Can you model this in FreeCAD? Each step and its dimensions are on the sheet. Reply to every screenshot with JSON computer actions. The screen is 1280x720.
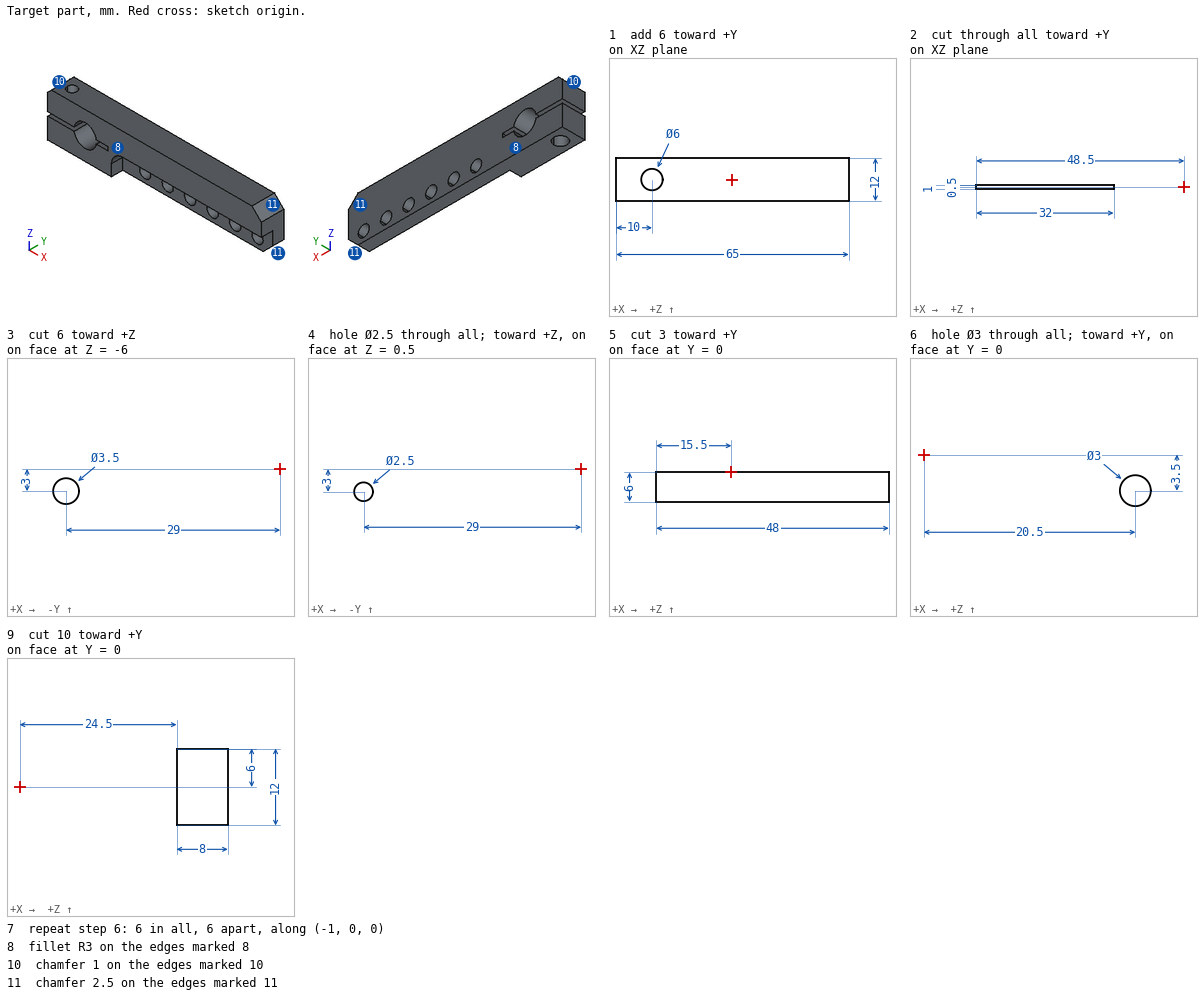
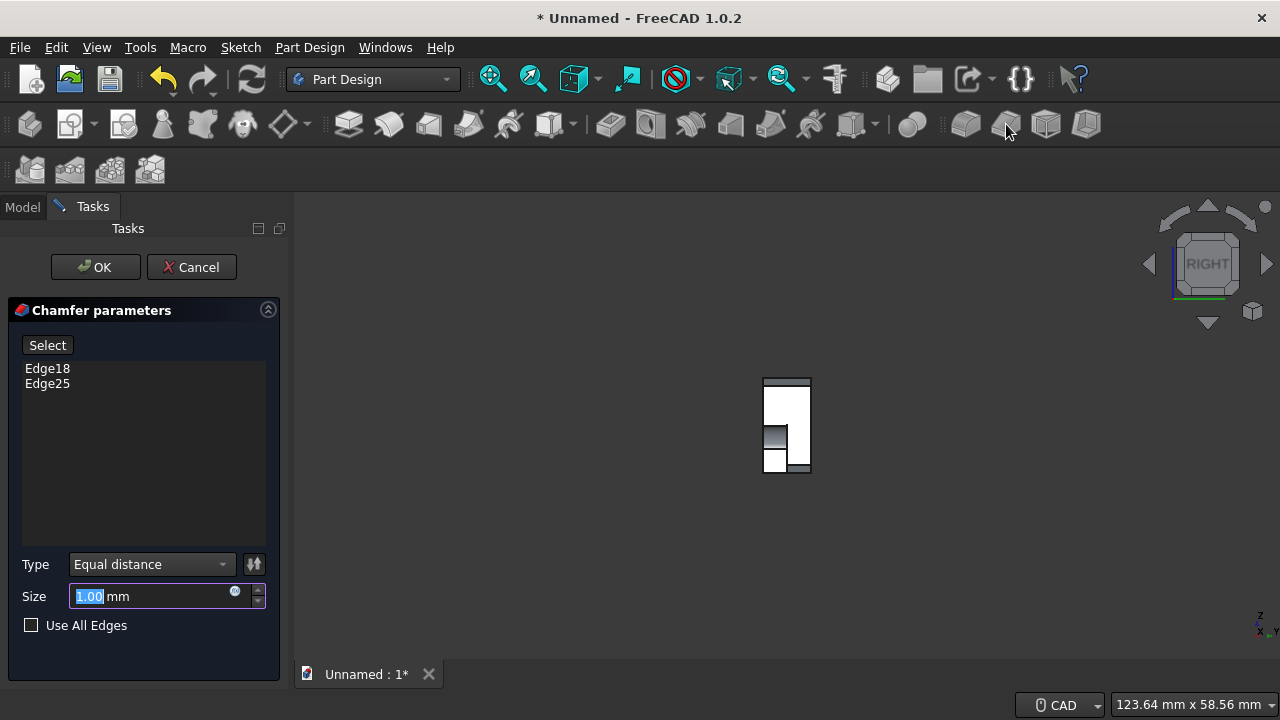
{"action": "type", "text": "2.5"}
{"action": "key", "text": "Tab"}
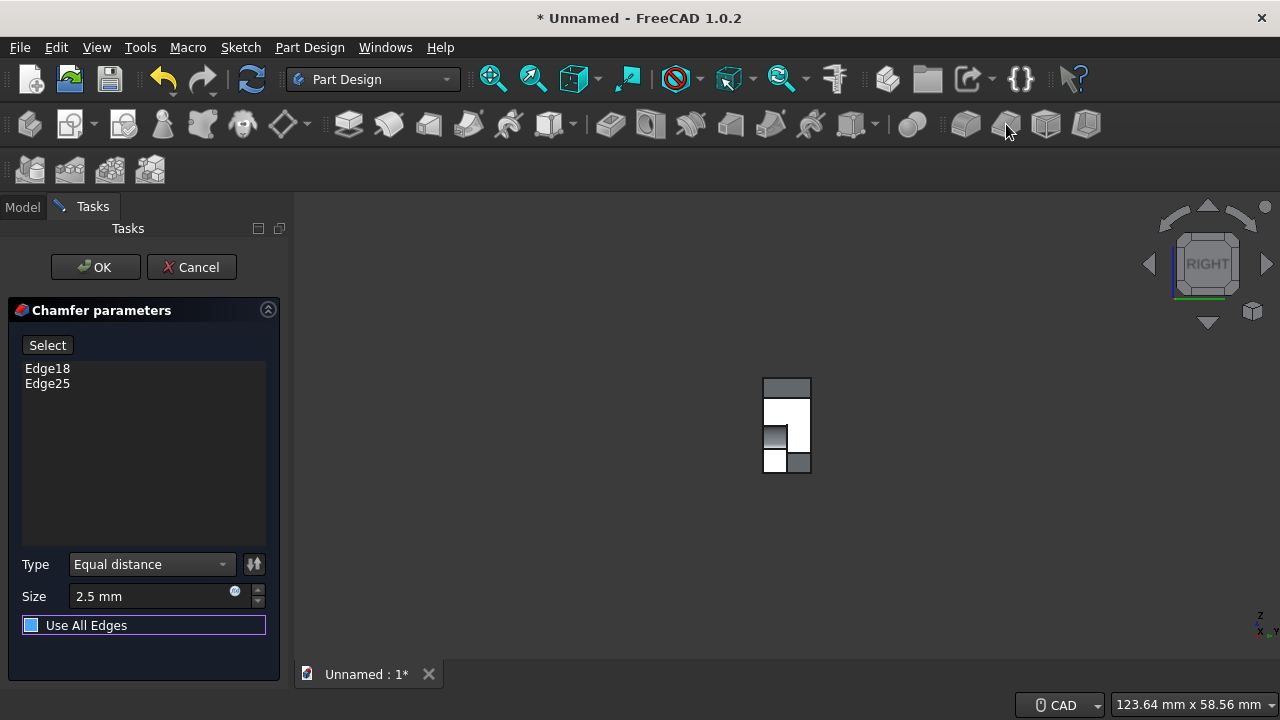
{"action": "left_click", "coordinate": [96, 267]}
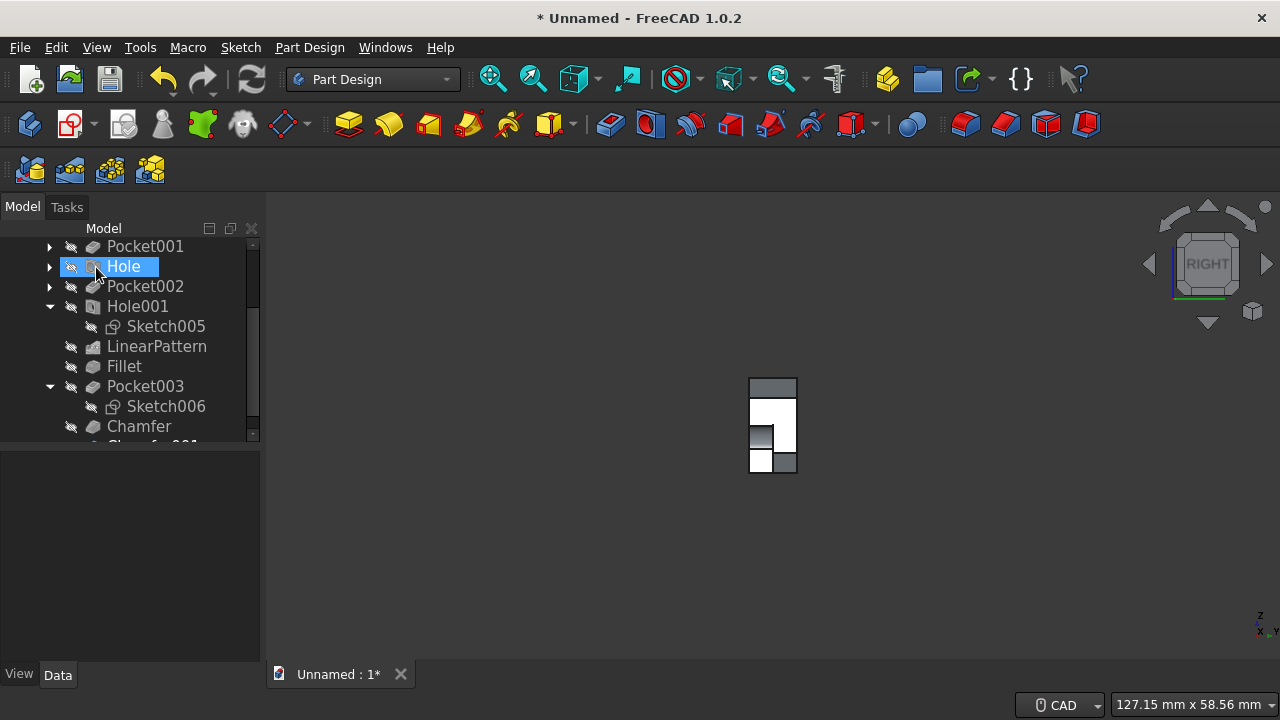
{"action": "key", "text": "0"}